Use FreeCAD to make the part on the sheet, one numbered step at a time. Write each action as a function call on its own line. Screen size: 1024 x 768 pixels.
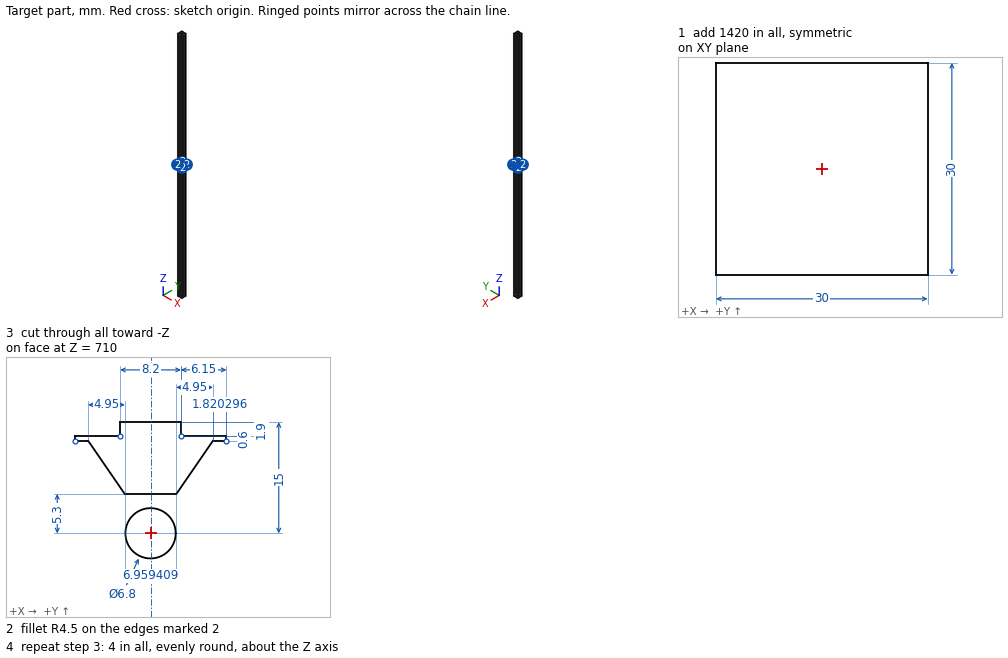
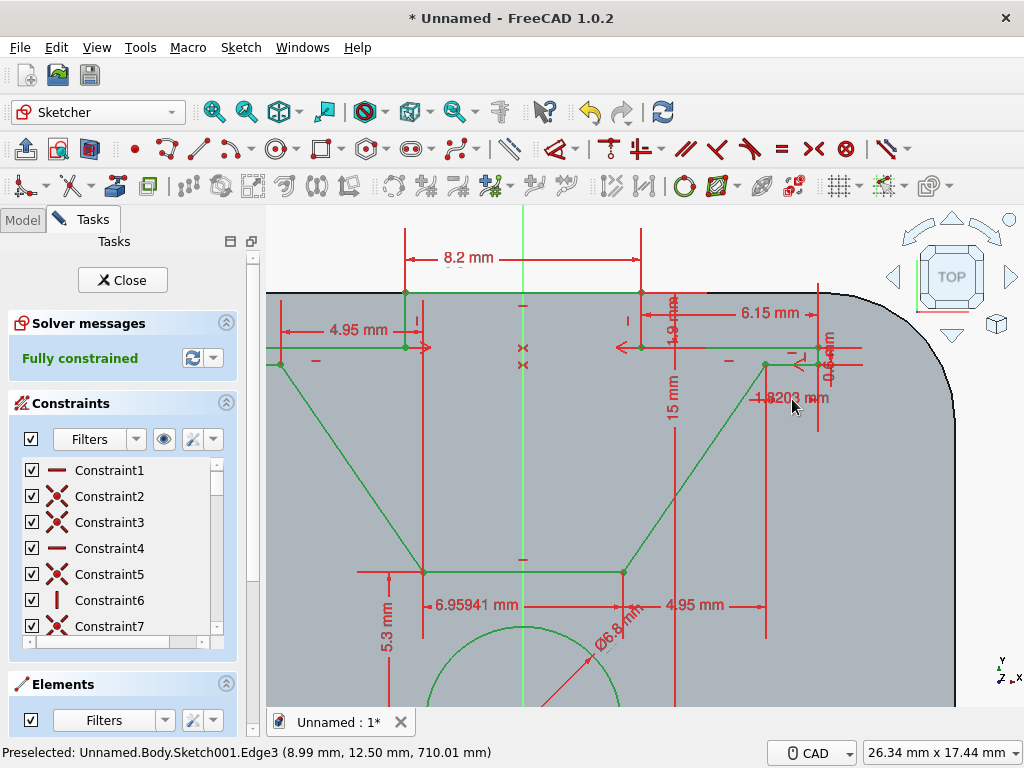
click(123, 280)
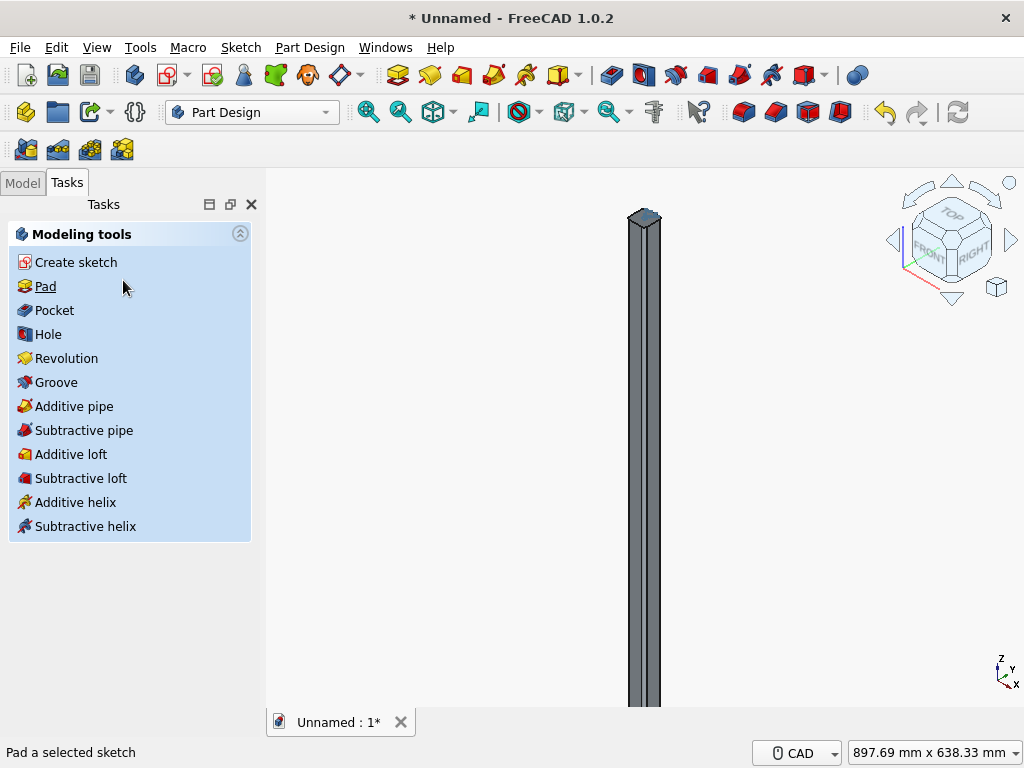
click(612, 76)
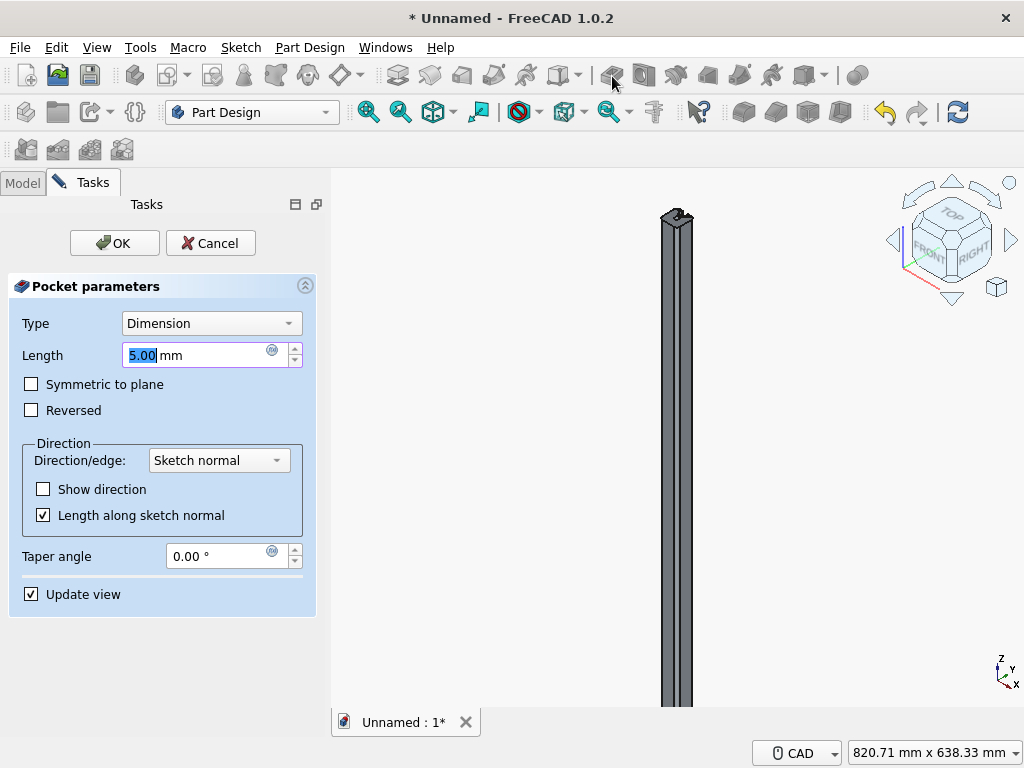
click(212, 324)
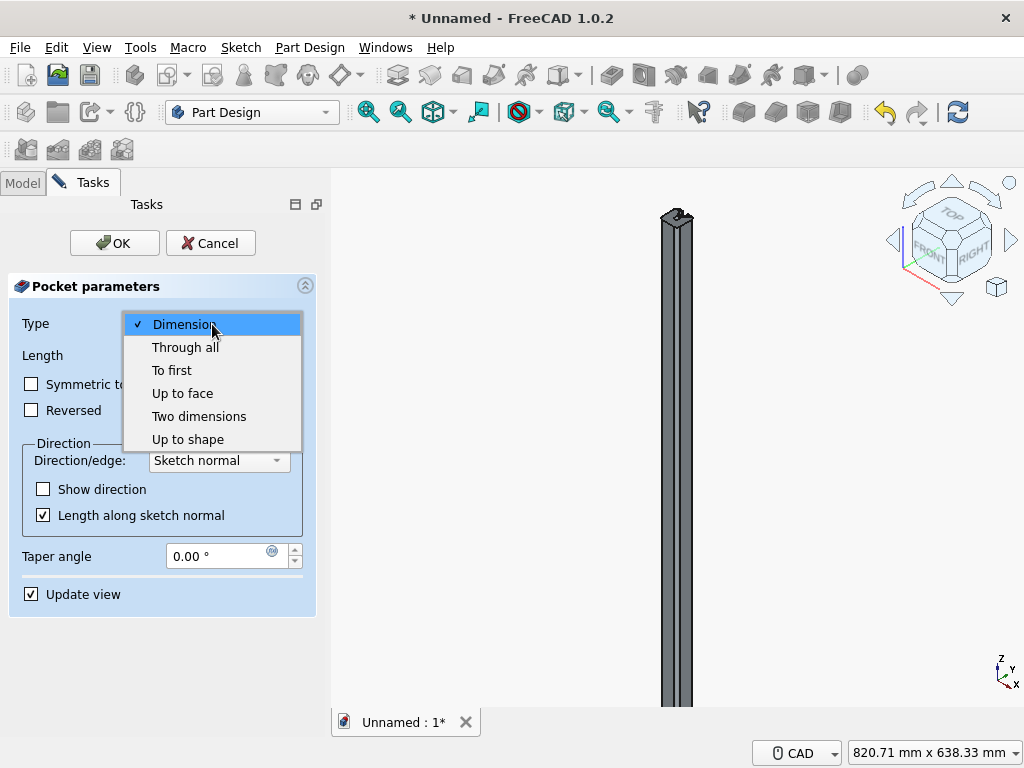
click(212, 348)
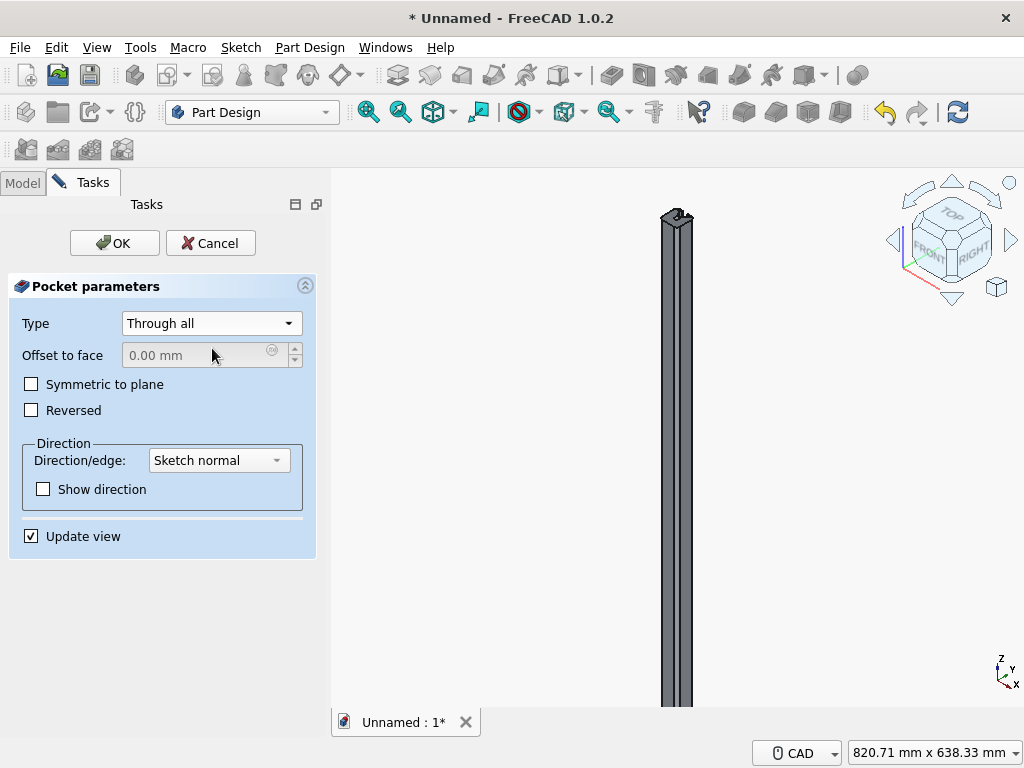
click(115, 243)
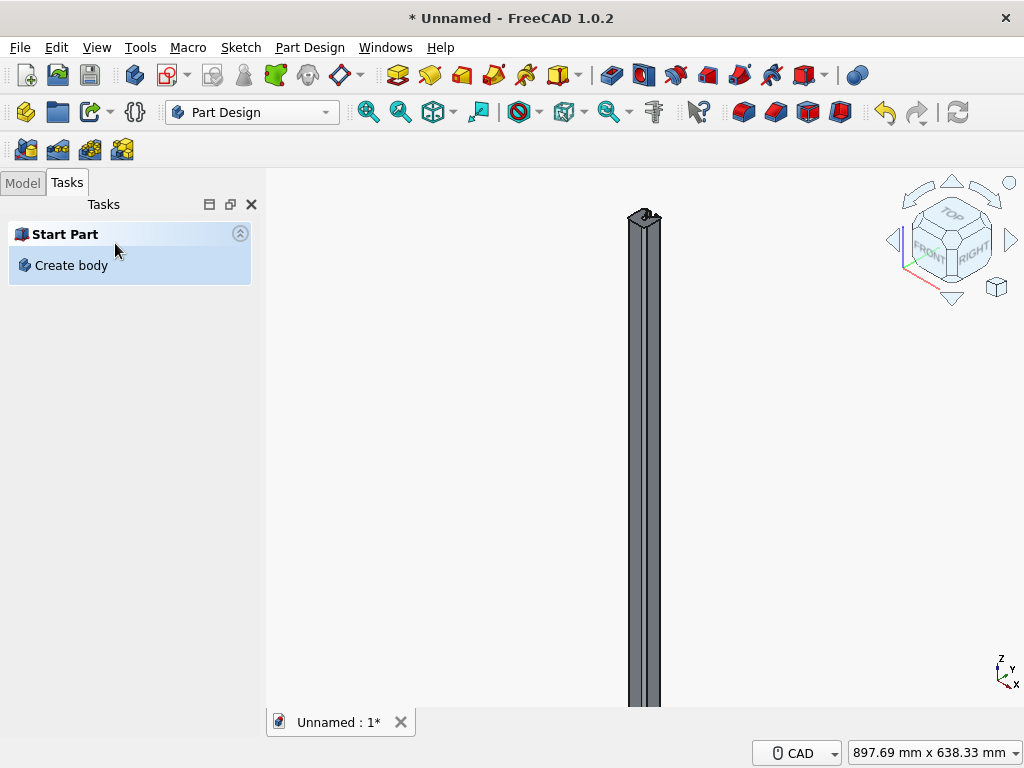
key(v)
key(f)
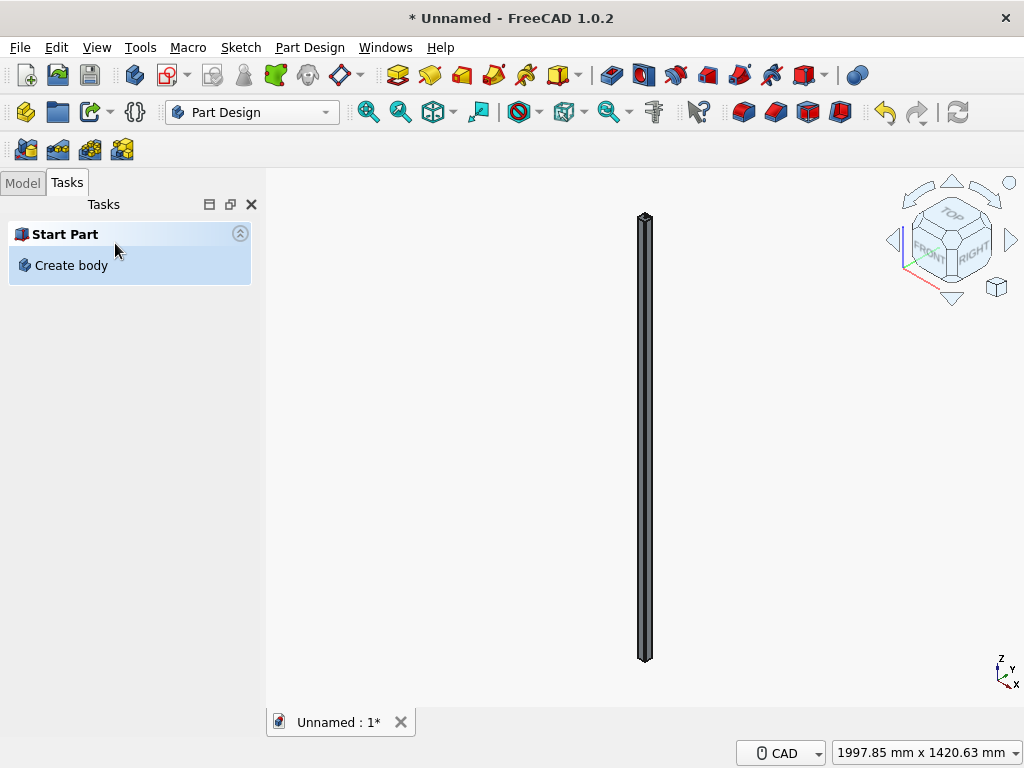
click(23, 182)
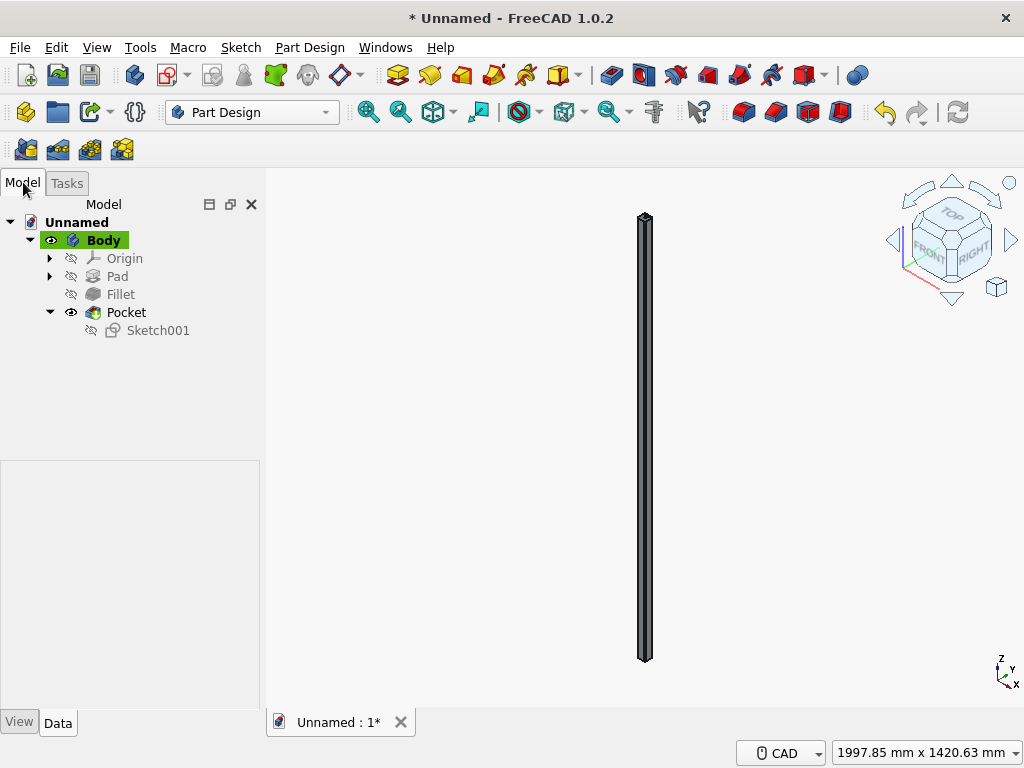
click(116, 312)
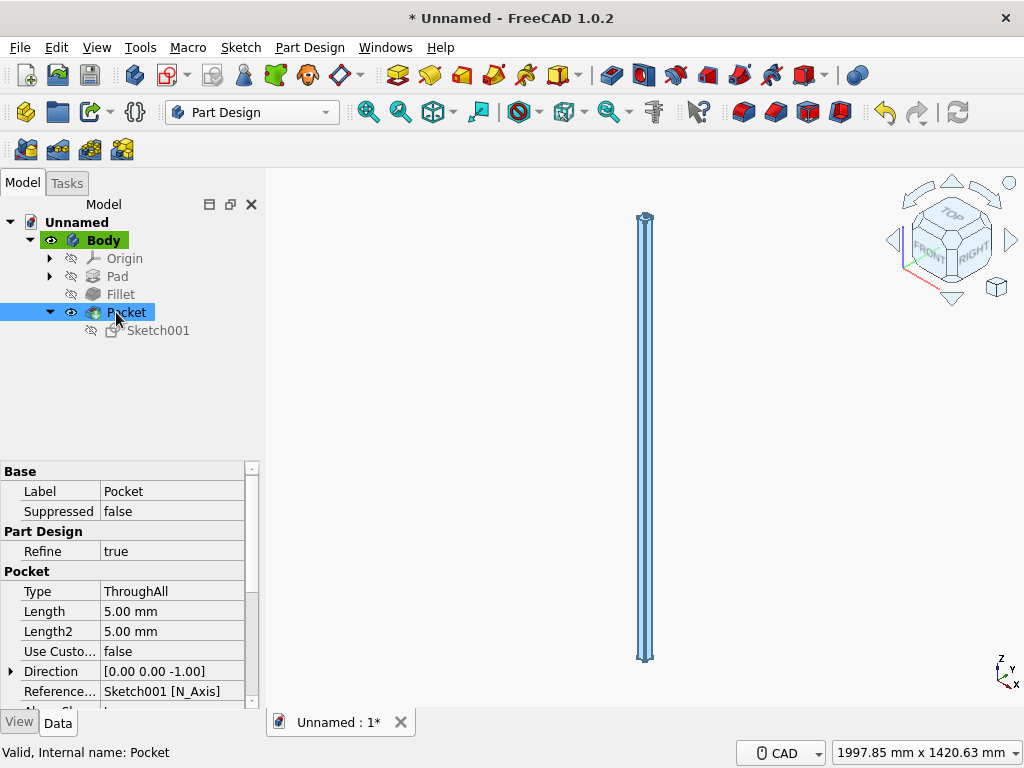
click(90, 150)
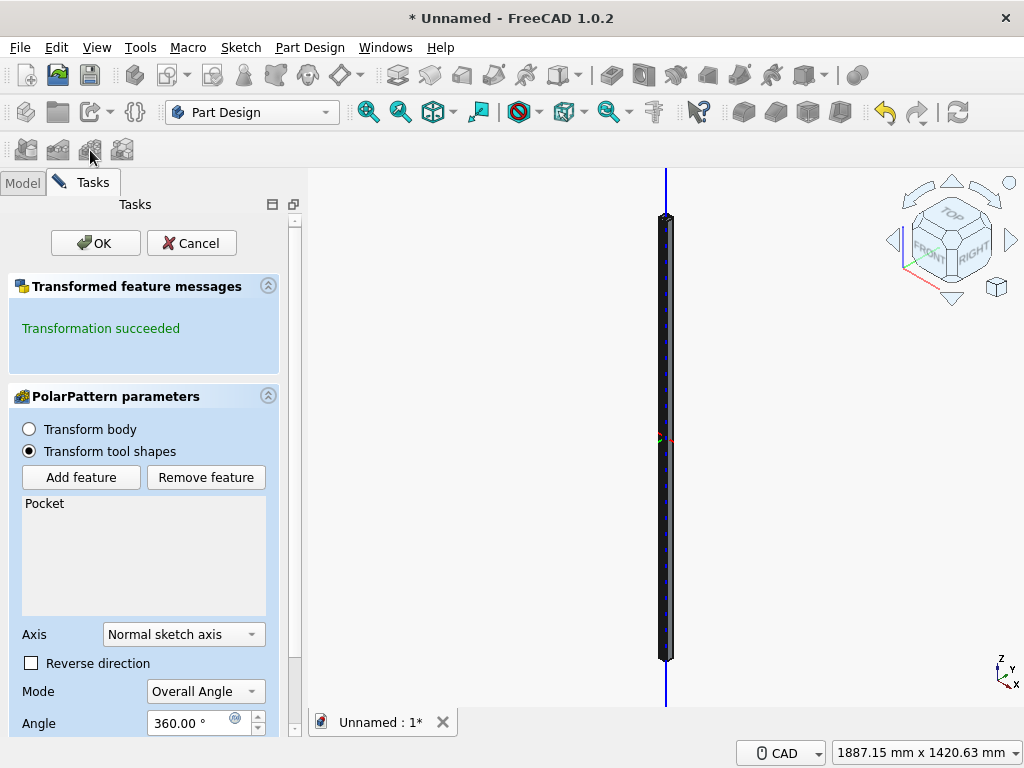
click(184, 634)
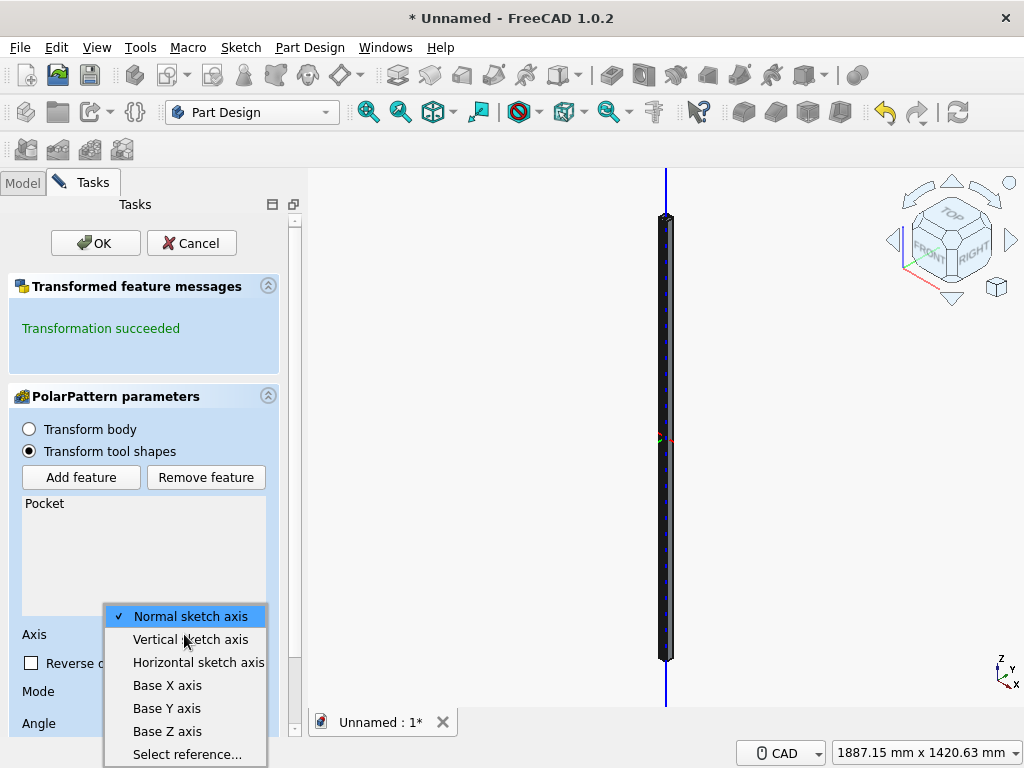
click(184, 732)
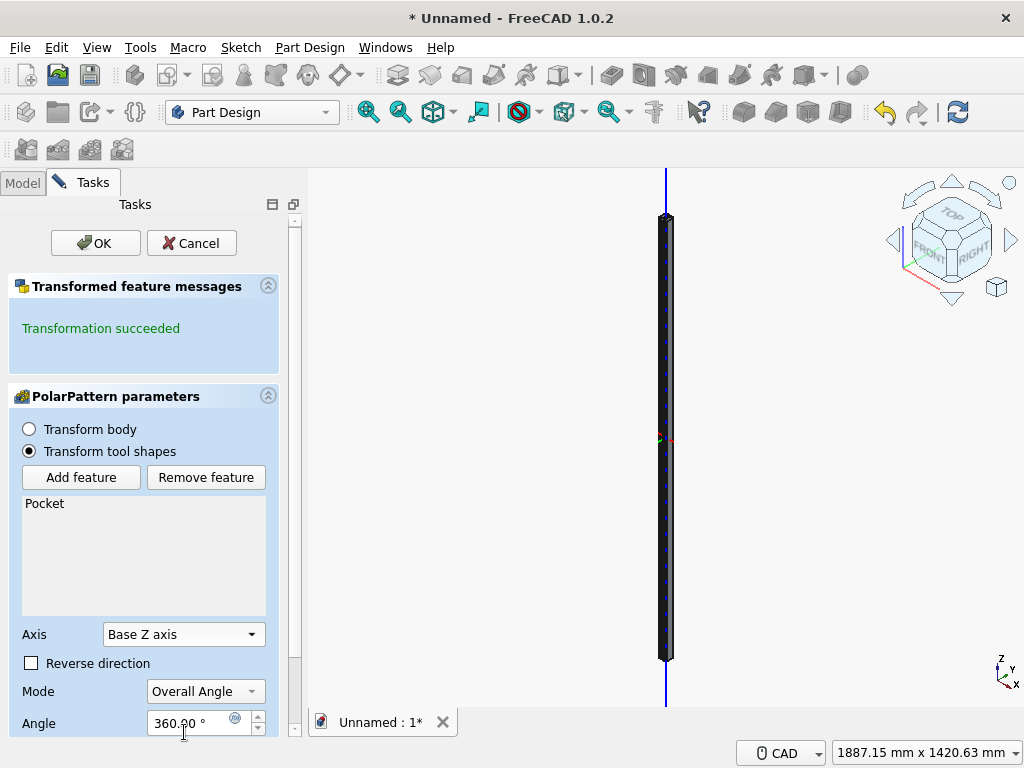
scroll(295, 475, down, 2)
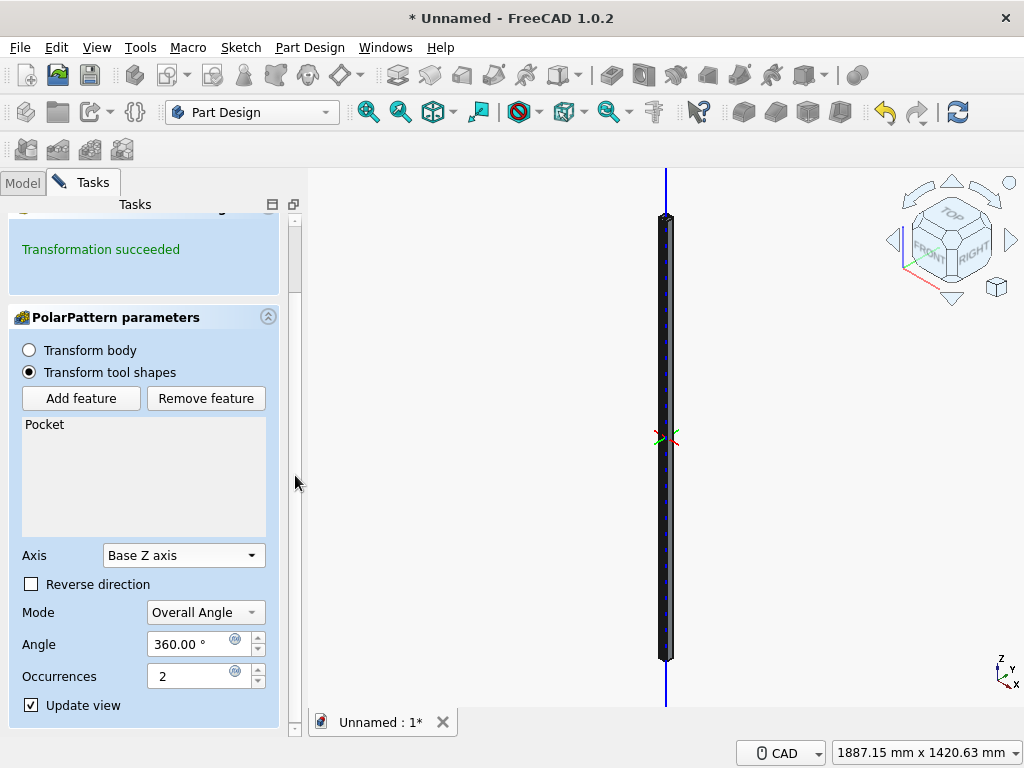
triple_click(198, 676)